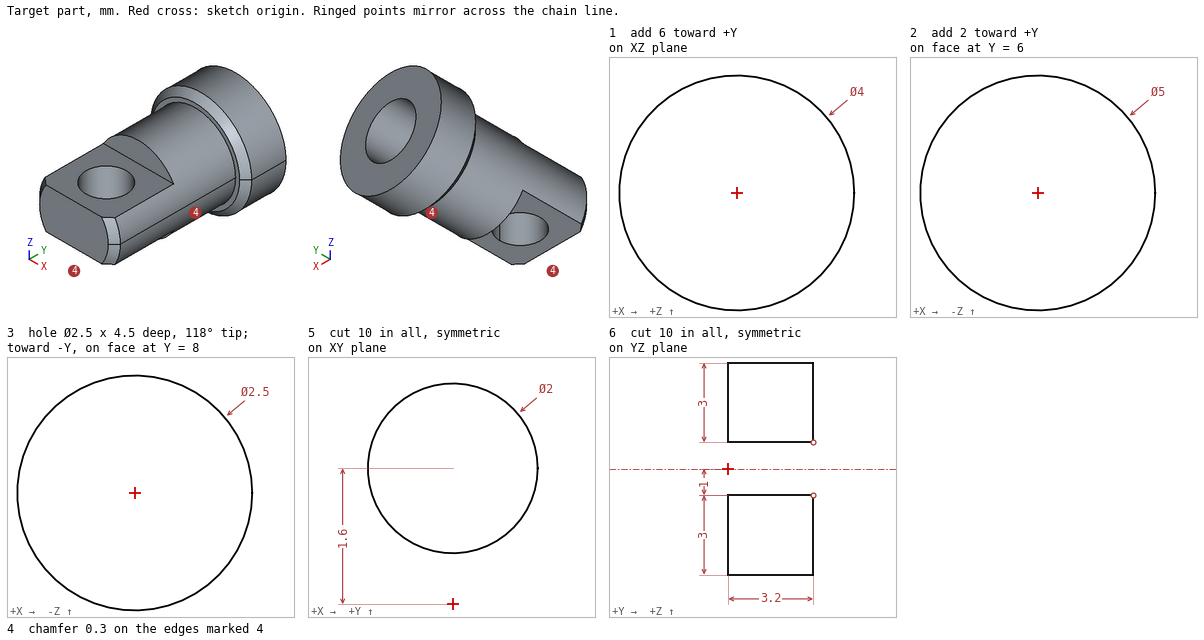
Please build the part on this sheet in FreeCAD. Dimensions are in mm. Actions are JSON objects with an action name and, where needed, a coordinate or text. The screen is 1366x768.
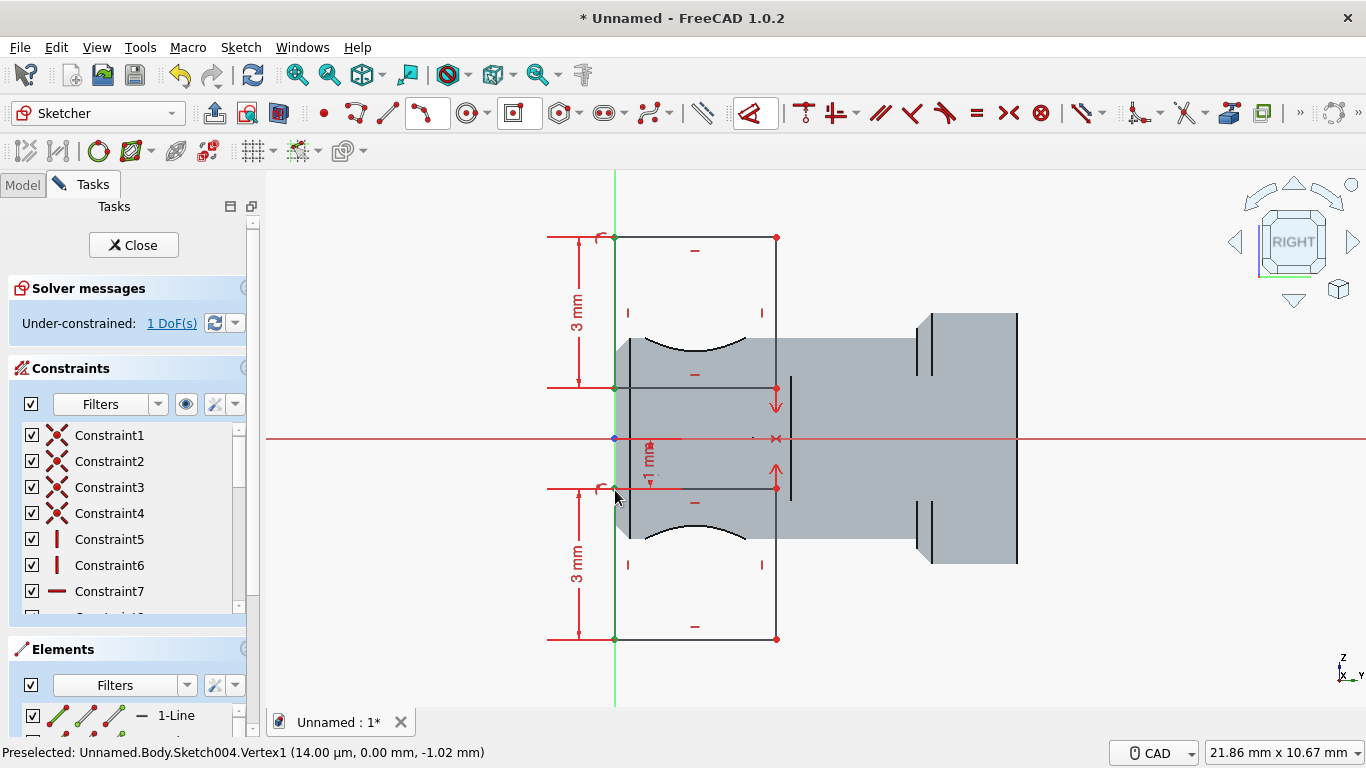
{"action": "left_click", "coordinate": [663, 640]}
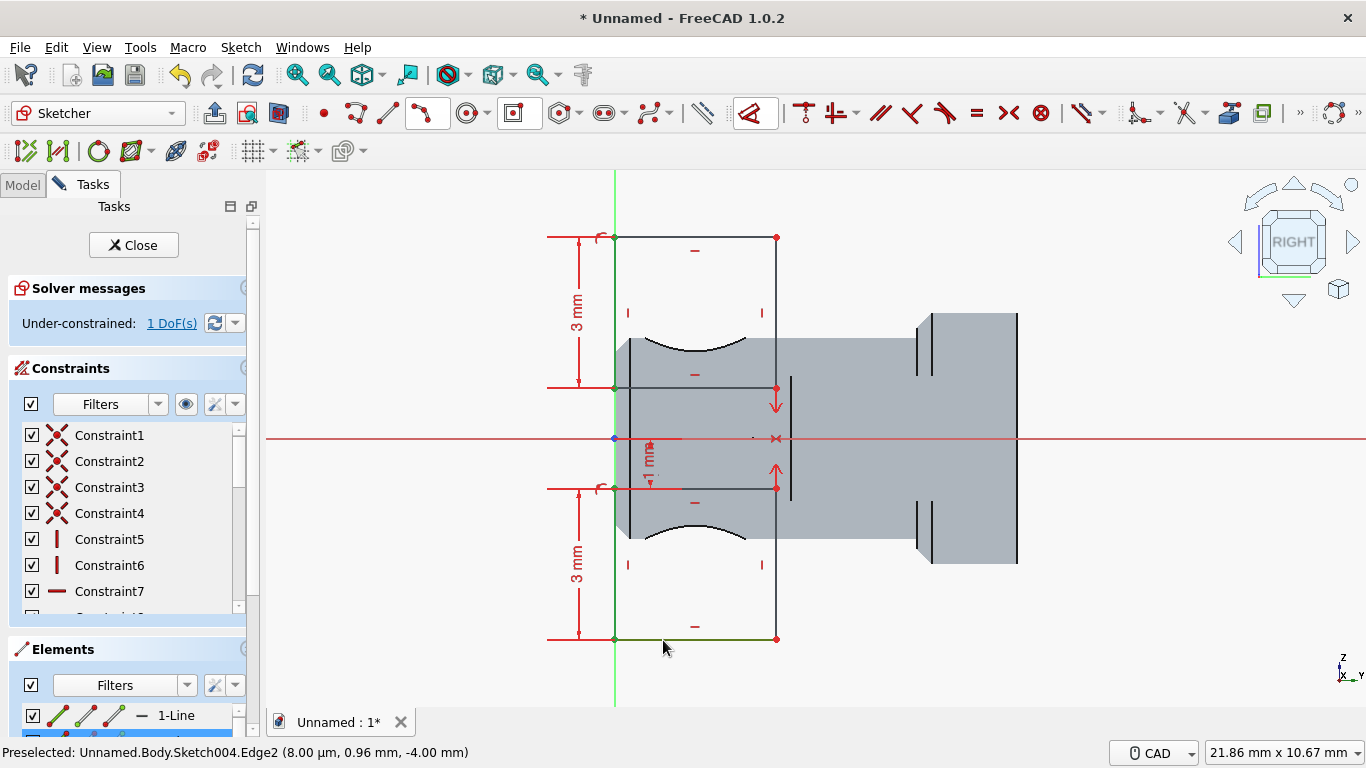
{"action": "key", "text": "l"}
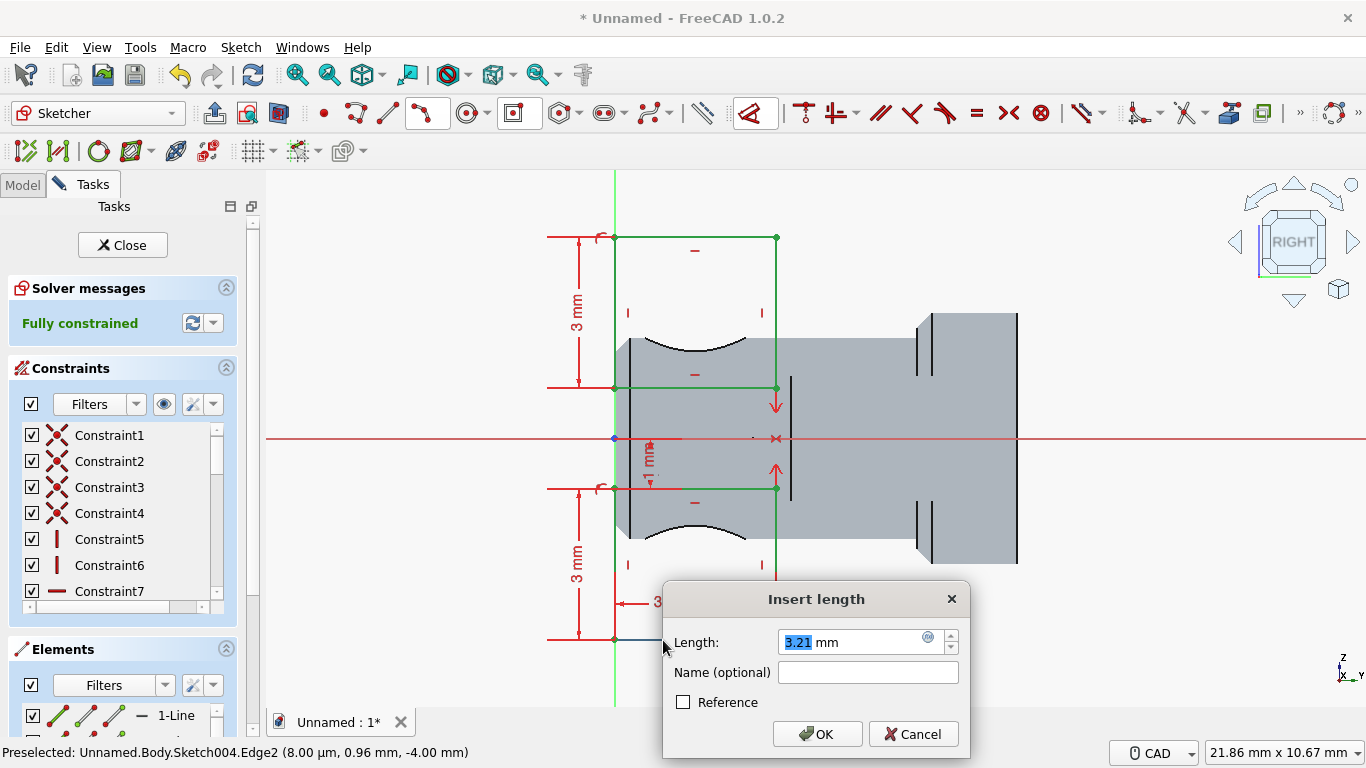
{"action": "type", "text": "3.2"}
{"action": "key", "text": "Return"}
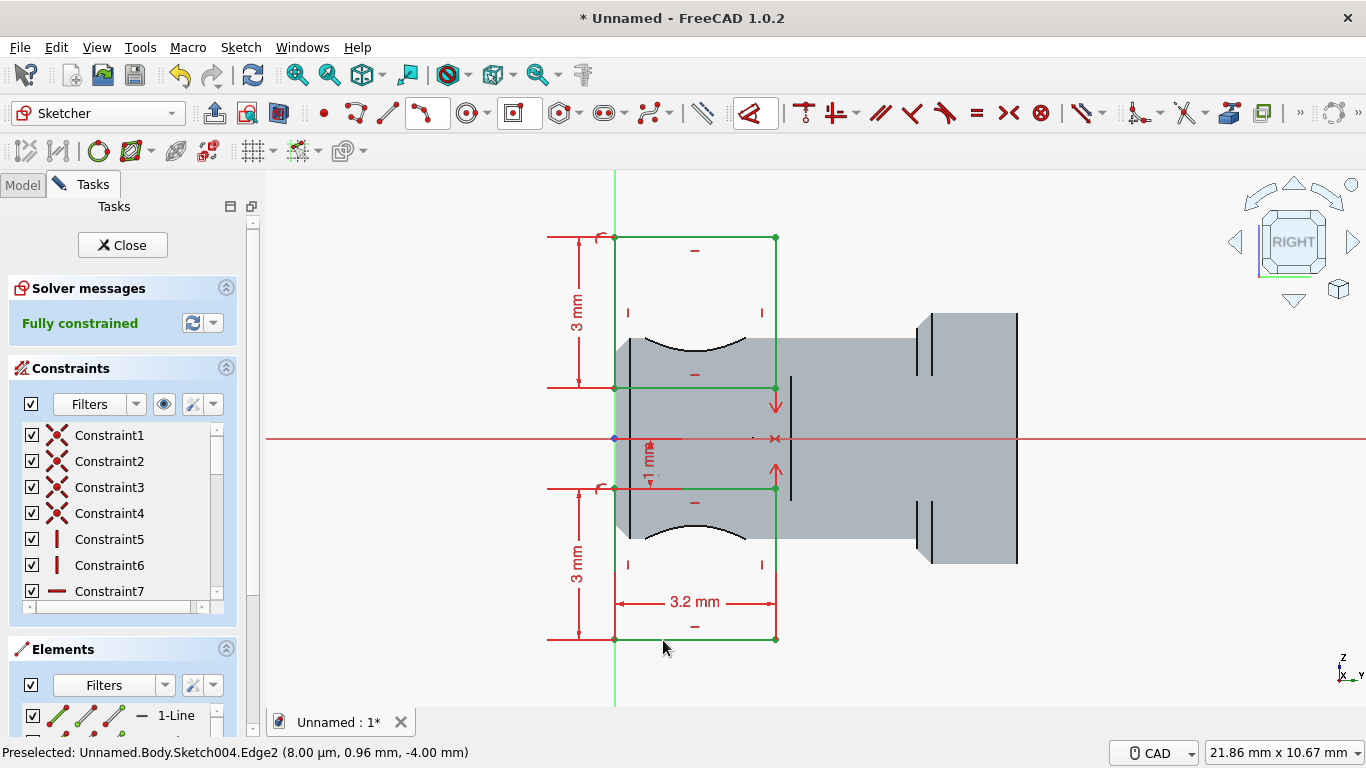
{"action": "left_click", "coordinate": [123, 245]}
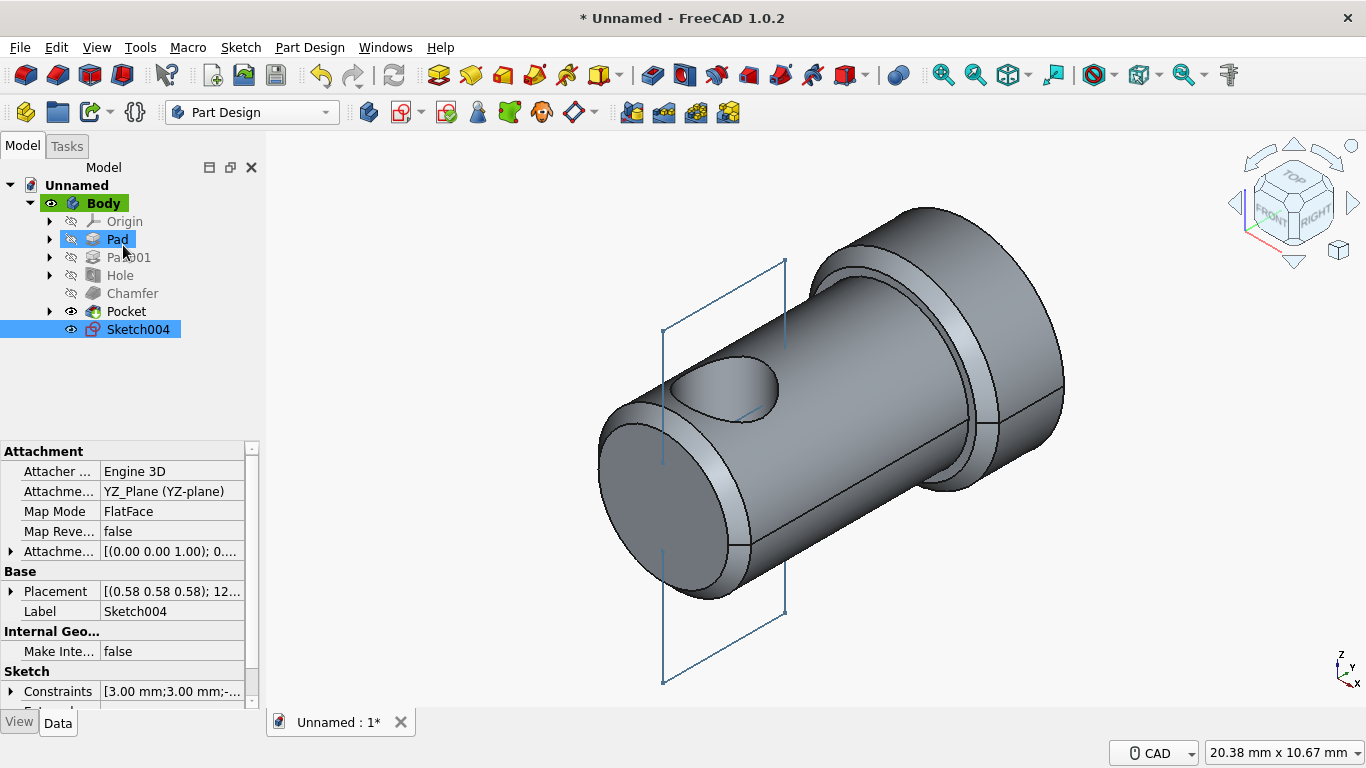
{"action": "left_click", "coordinate": [654, 76]}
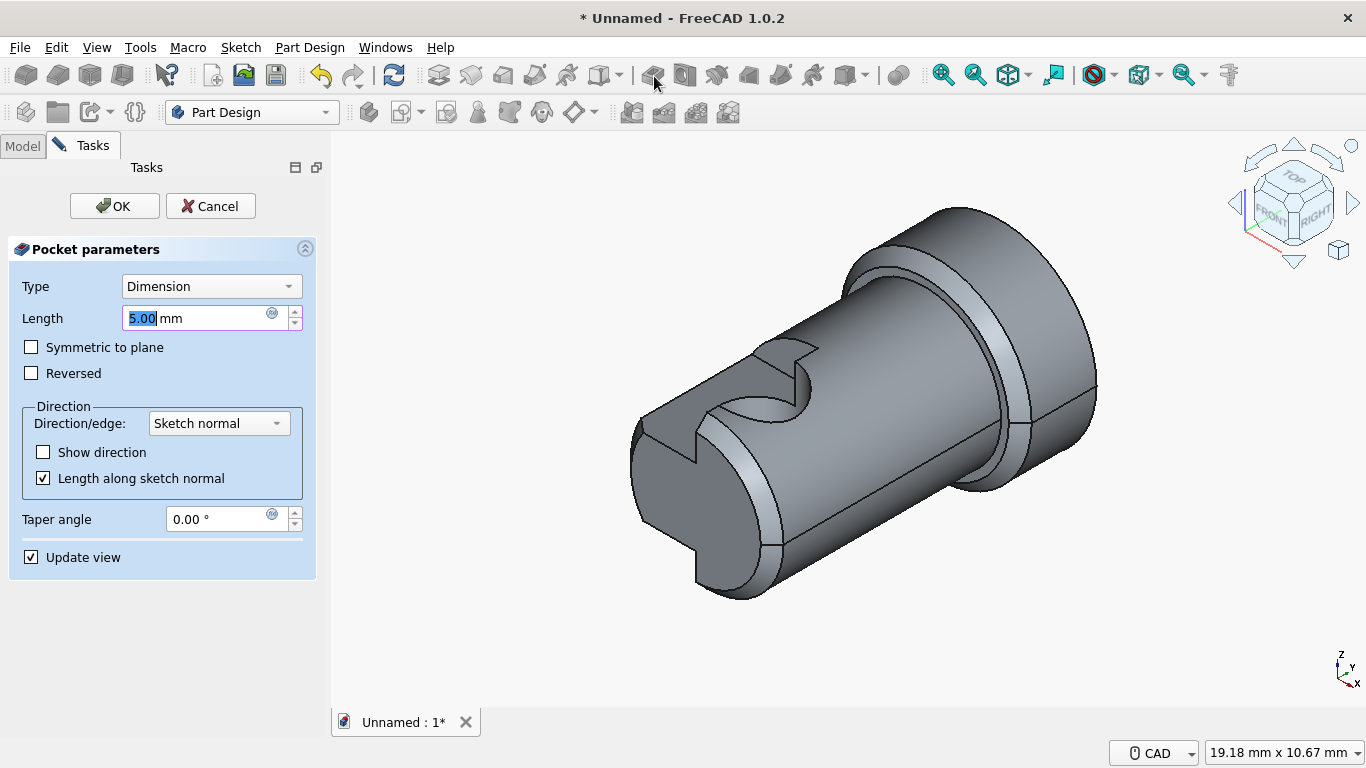
{"action": "type", "text": "10"}
{"action": "key", "text": "Tab"}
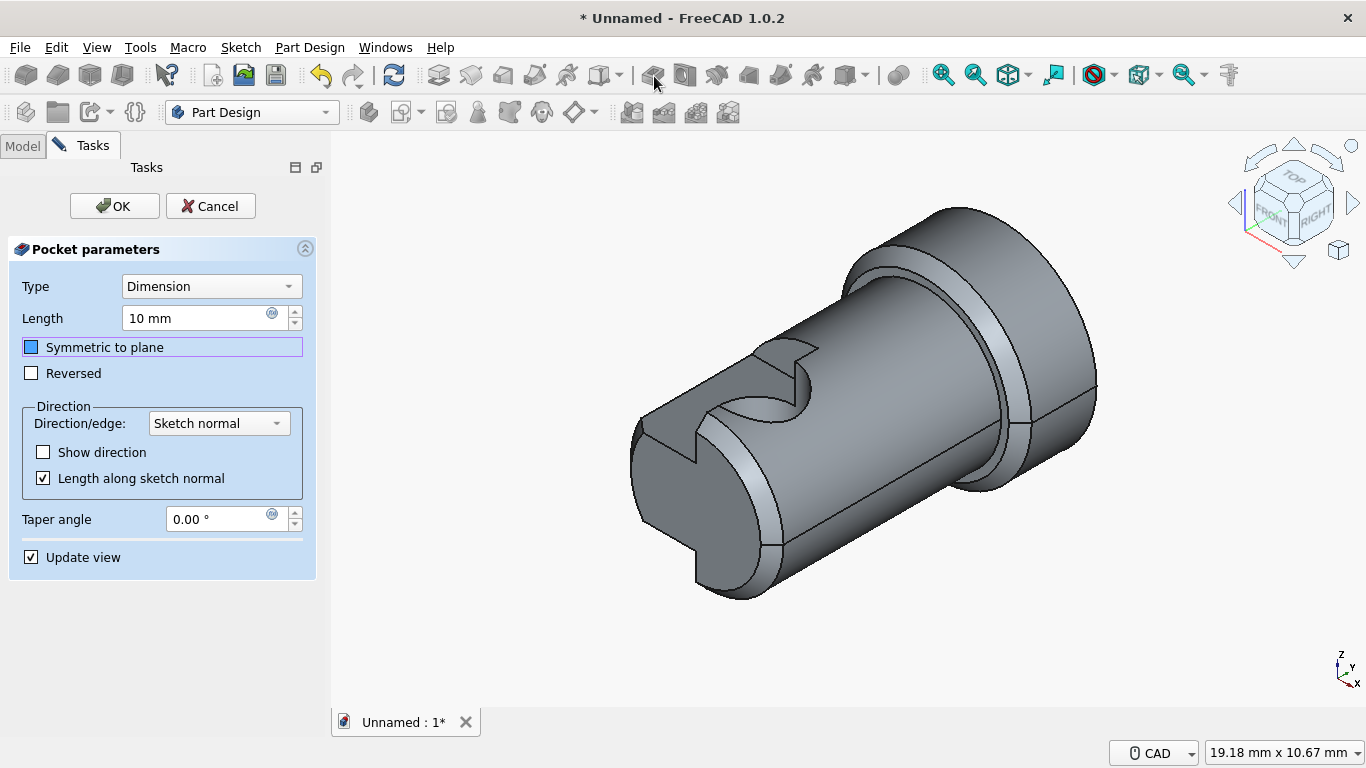
{"action": "left_click", "coordinate": [30, 347]}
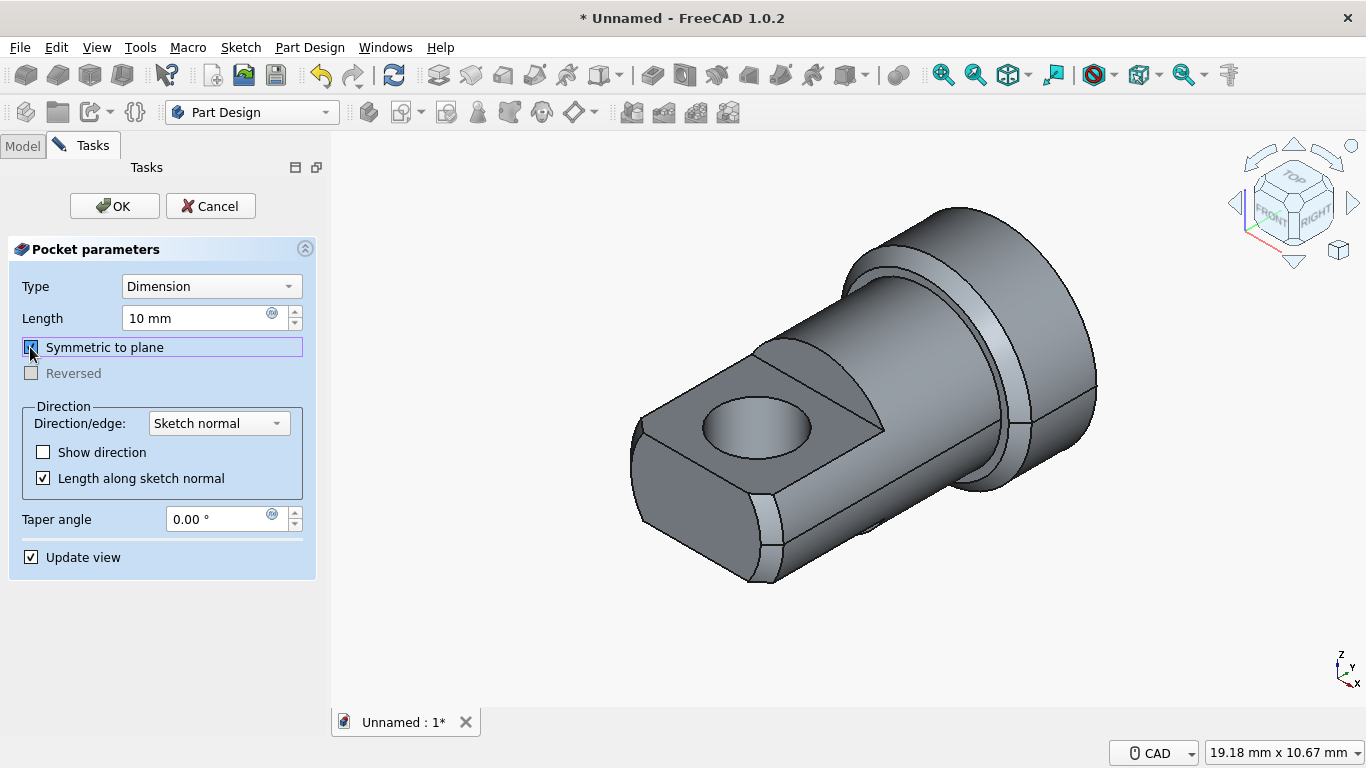
{"action": "left_click", "coordinate": [115, 206]}